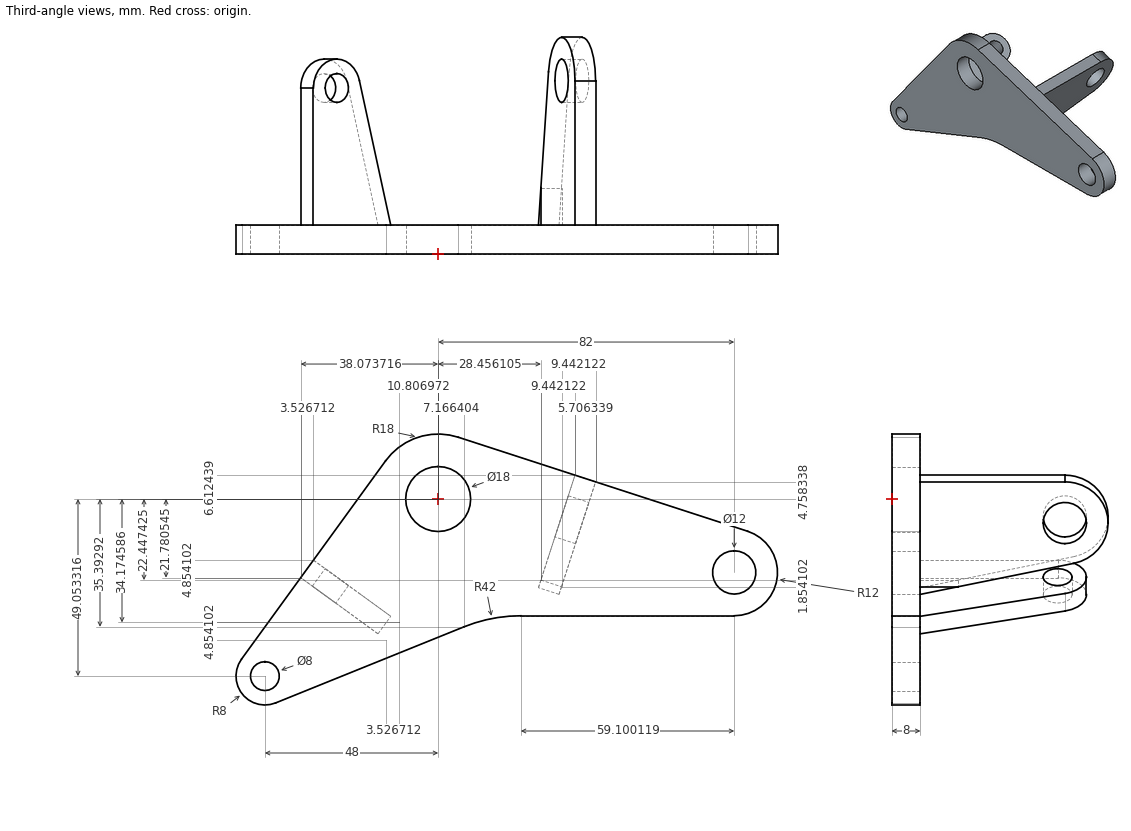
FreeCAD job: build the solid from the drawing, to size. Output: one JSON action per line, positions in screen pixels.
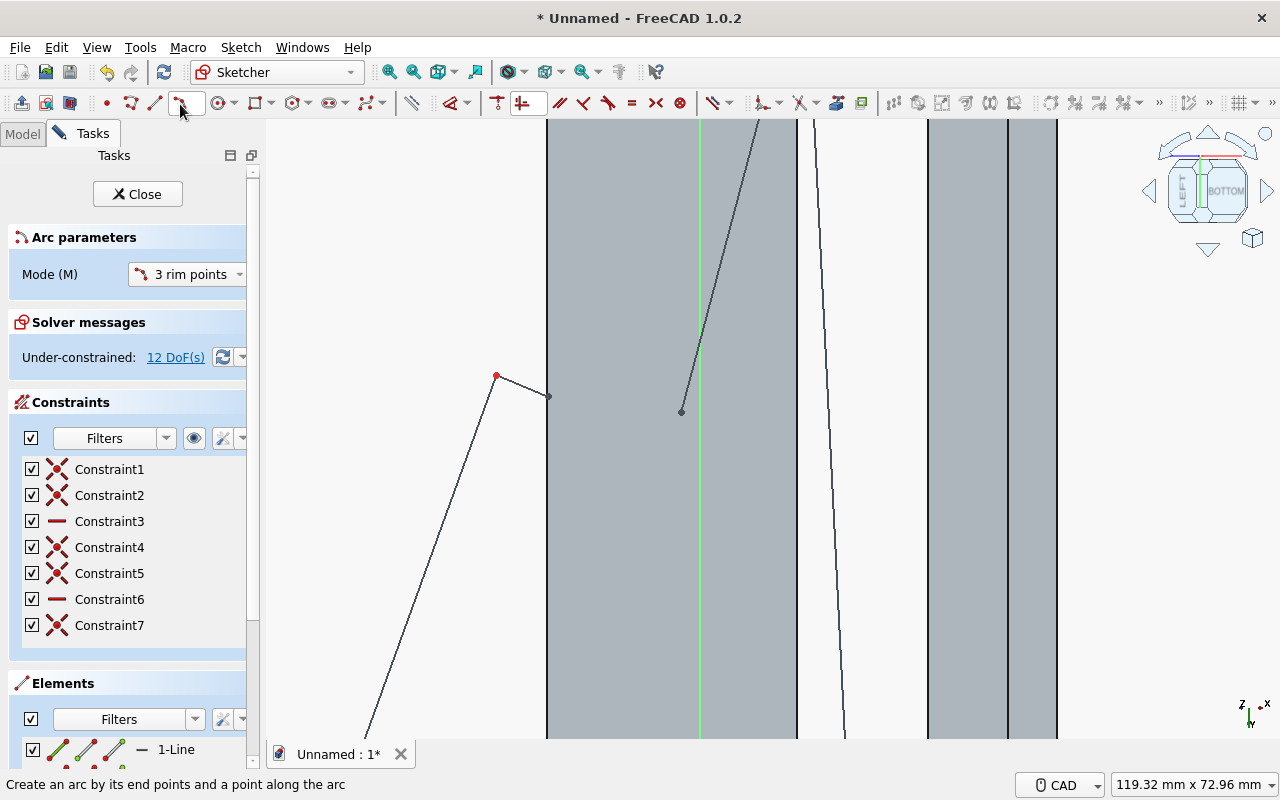
{"action": "left_click", "coordinate": [681, 413]}
{"action": "left_click", "coordinate": [548, 397]}
{"action": "left_click", "coordinate": [607, 462]}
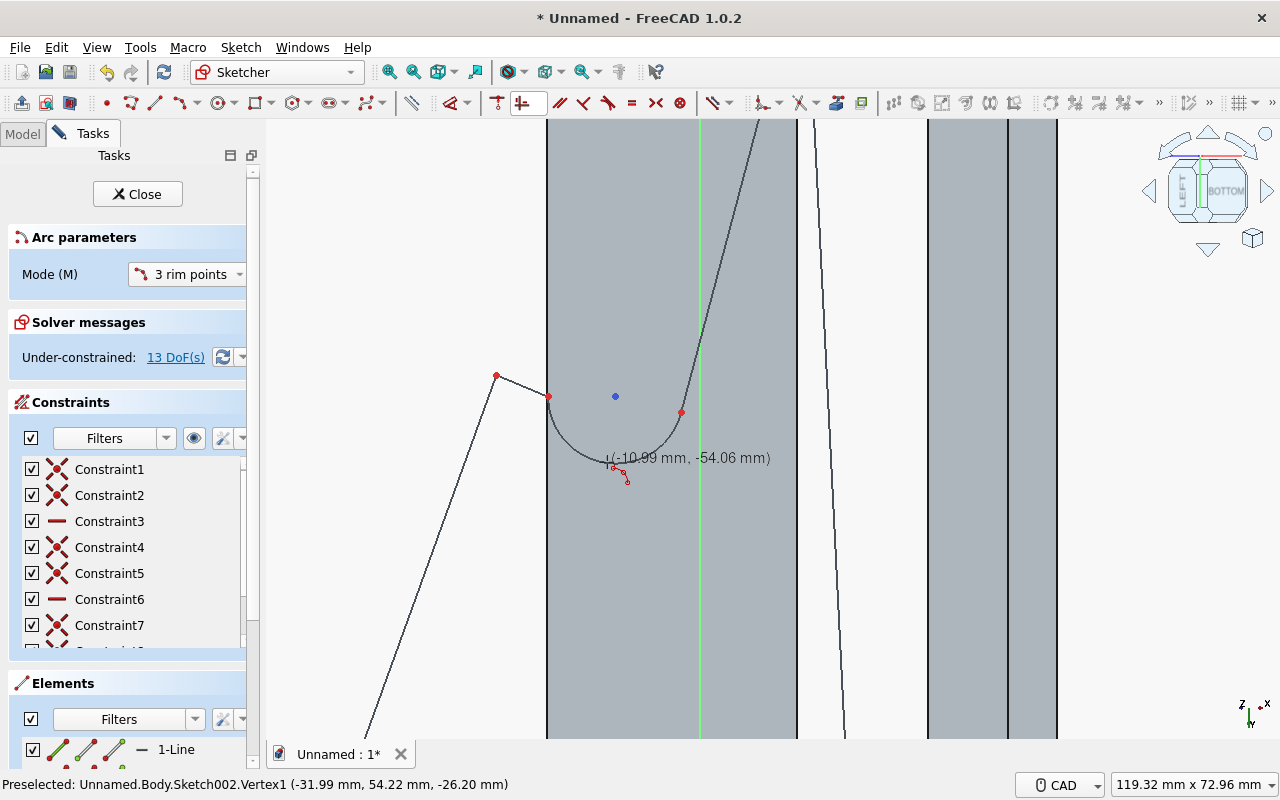
{"action": "left_click", "coordinate": [218, 104]}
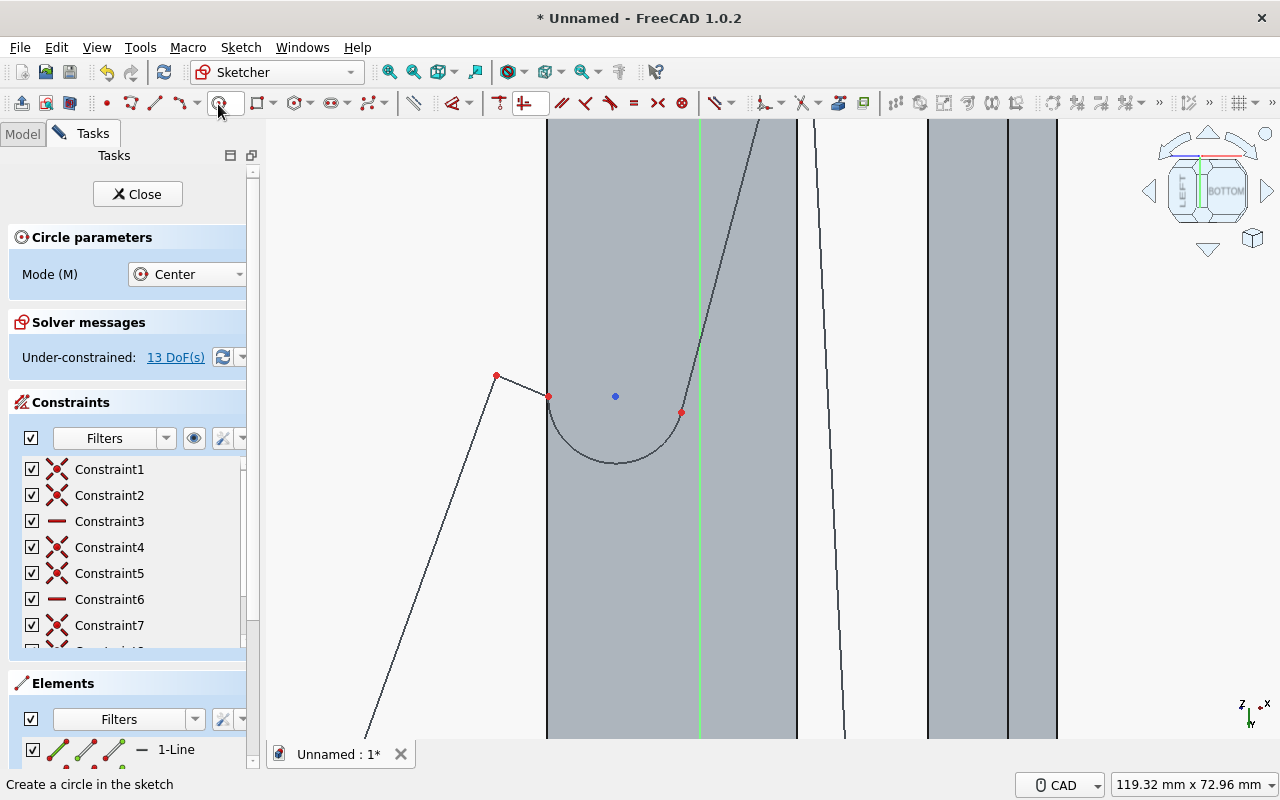
{"action": "left_click", "coordinate": [615, 394]}
{"action": "mouse_move", "coordinate": [639, 370]}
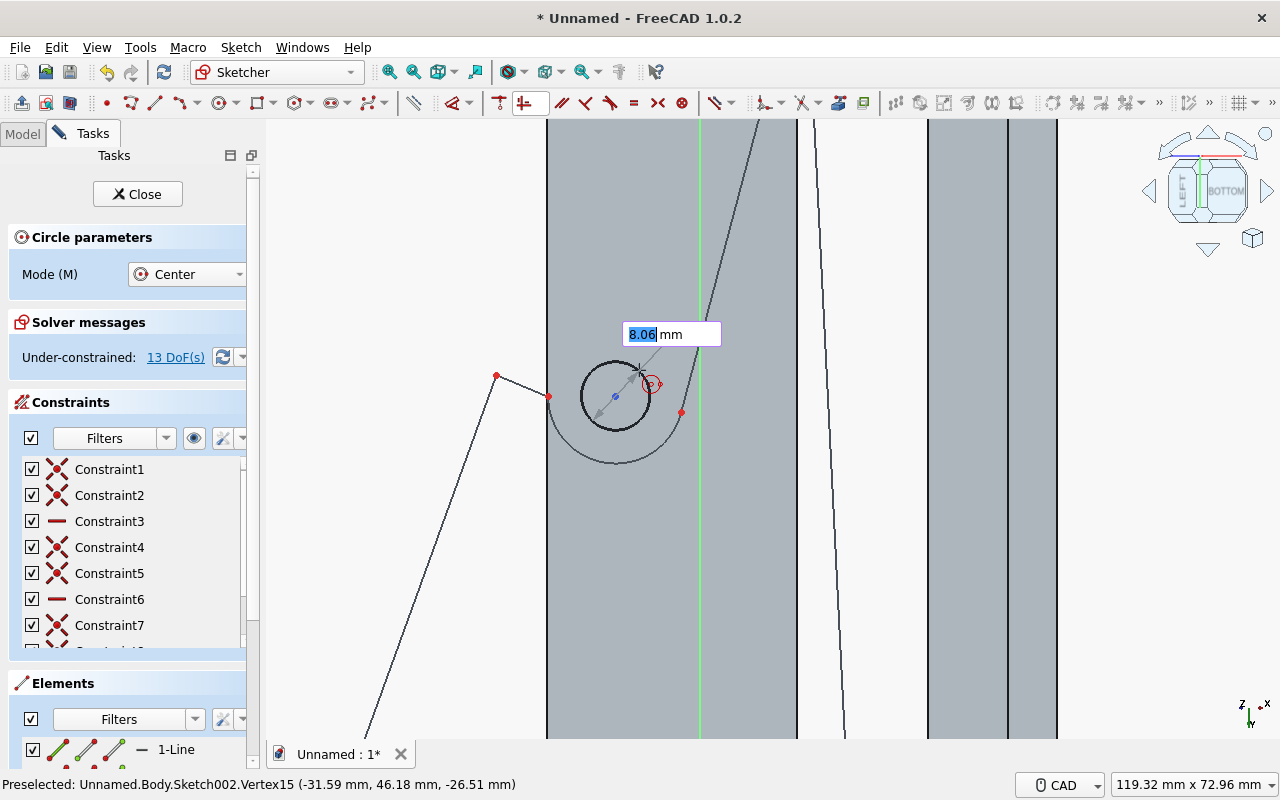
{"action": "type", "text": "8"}
{"action": "key", "text": "Return"}
{"action": "key", "text": "Escape"}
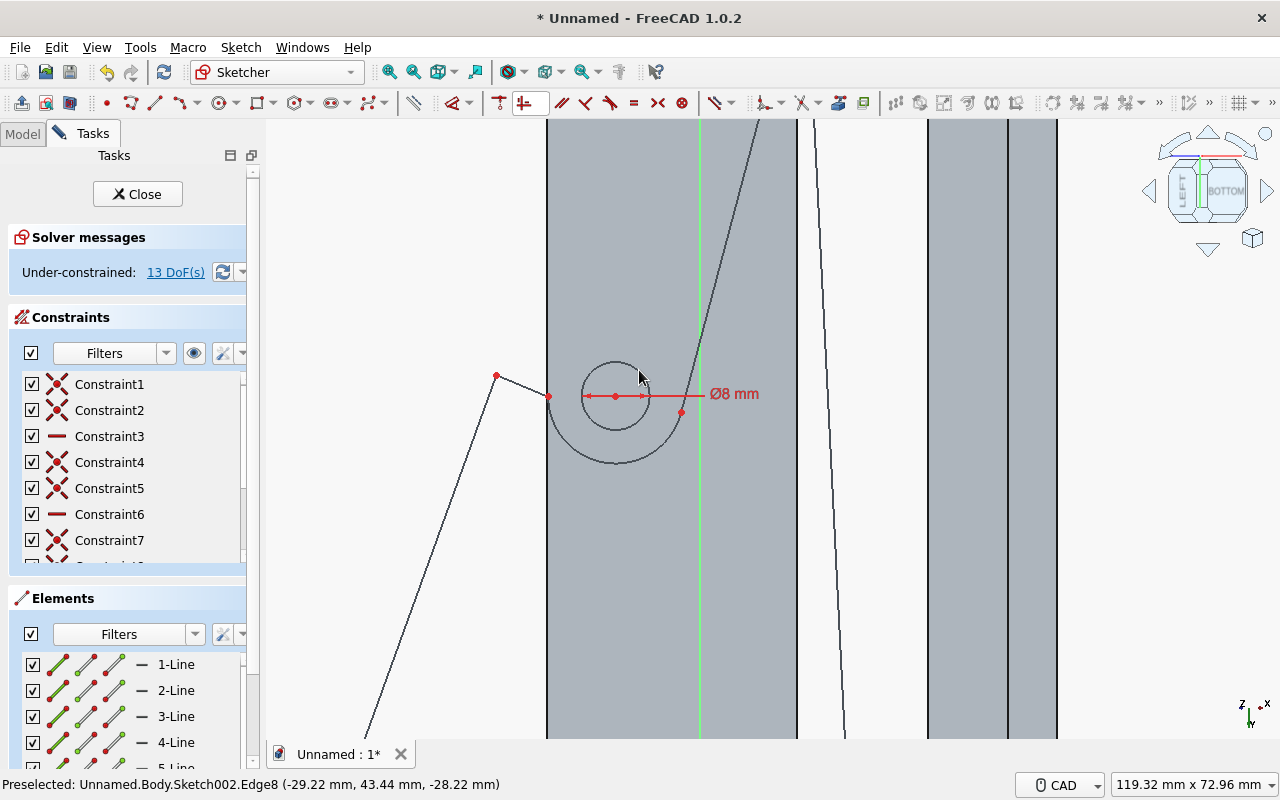
{"action": "left_click", "coordinate": [744, 175]}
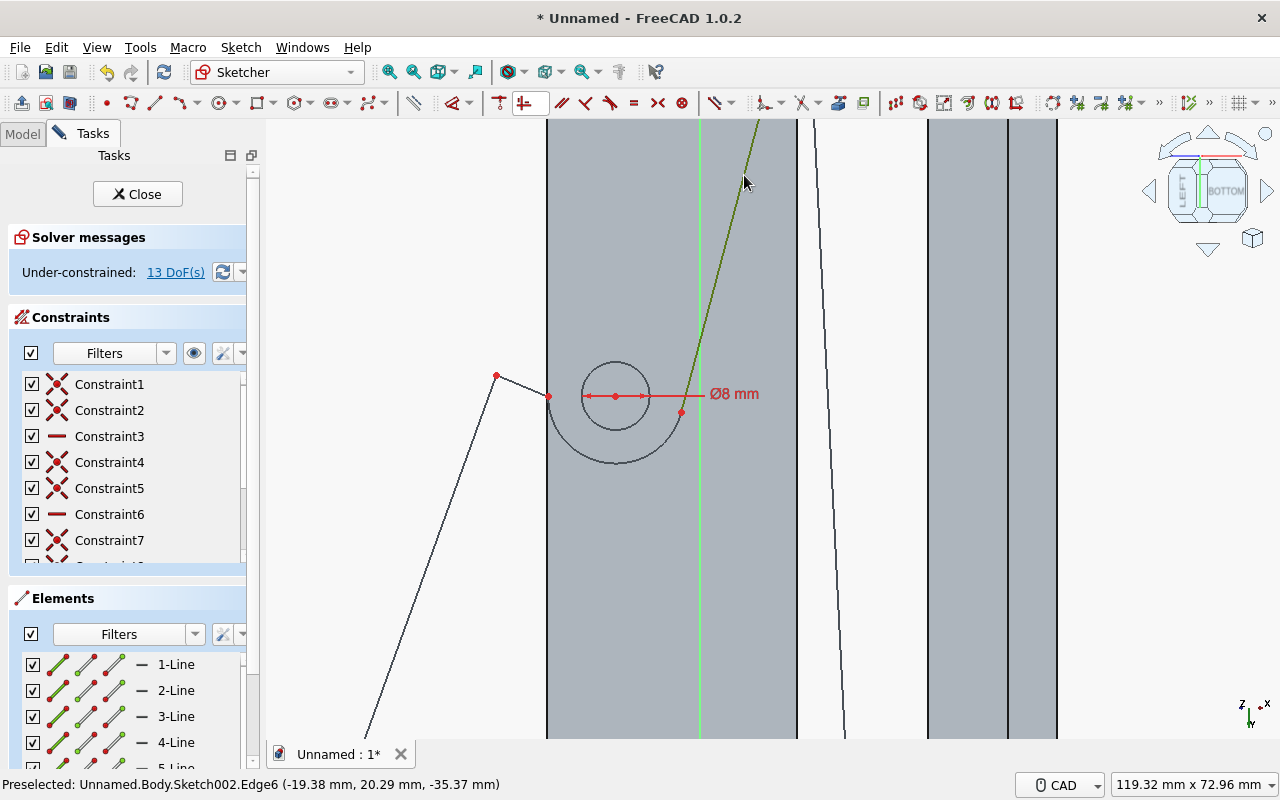
{"action": "left_click", "coordinate": [572, 448]}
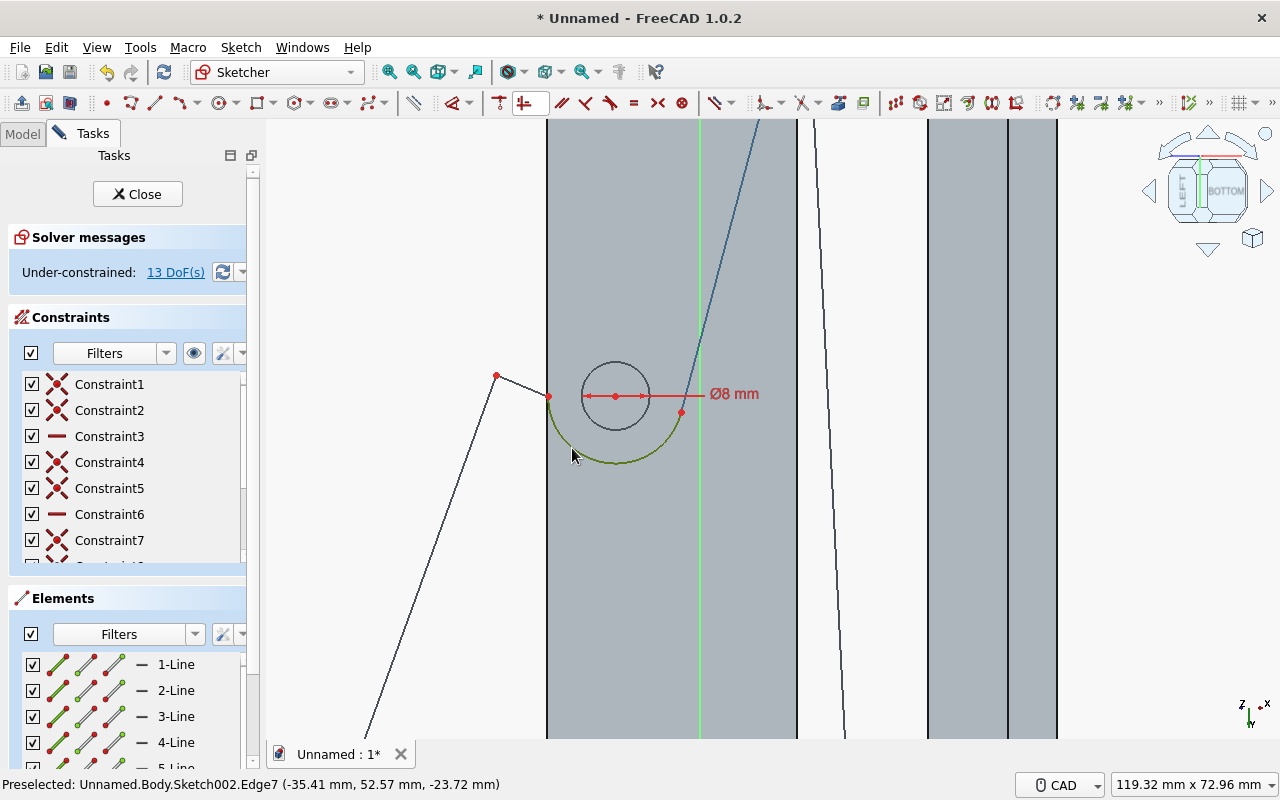
{"action": "left_click", "coordinate": [610, 104]}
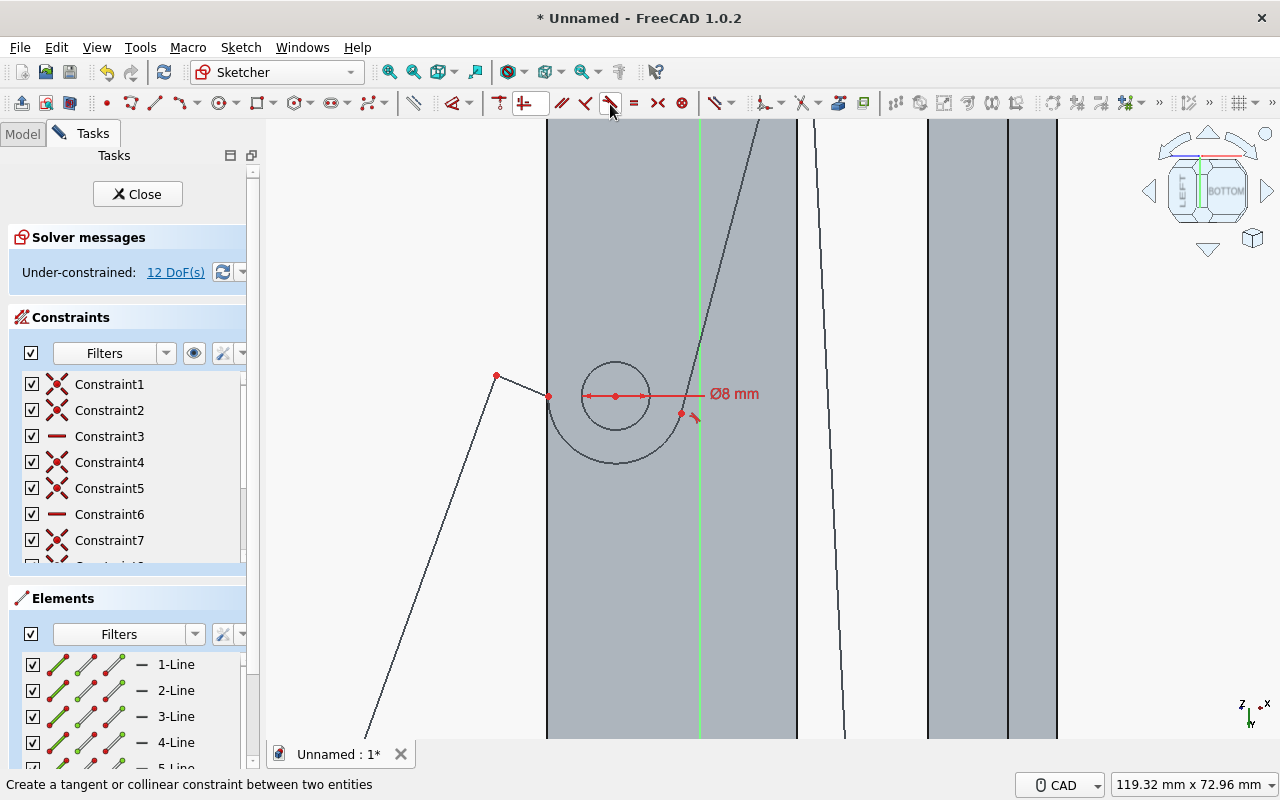
{"action": "left_click", "coordinate": [452, 104]}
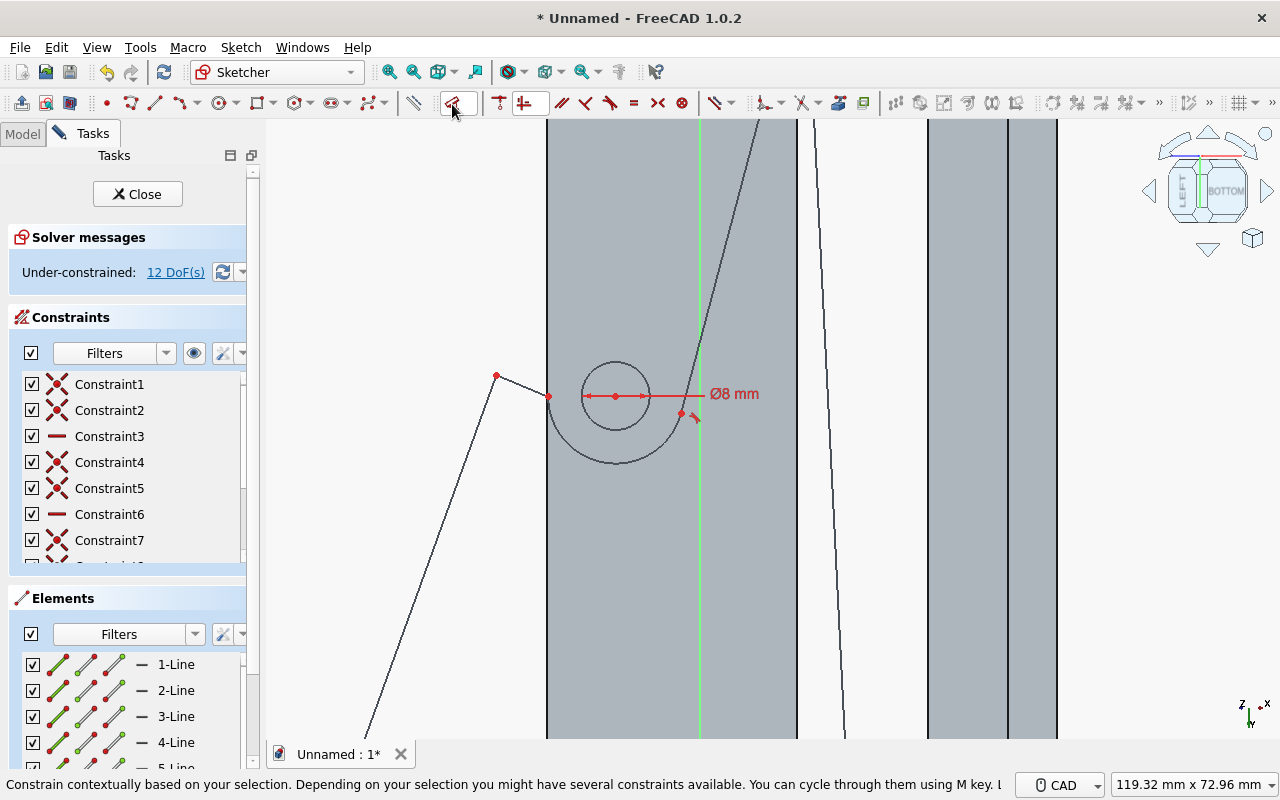
{"action": "left_click", "coordinate": [572, 448]}
{"action": "left_click", "coordinate": [551, 473]}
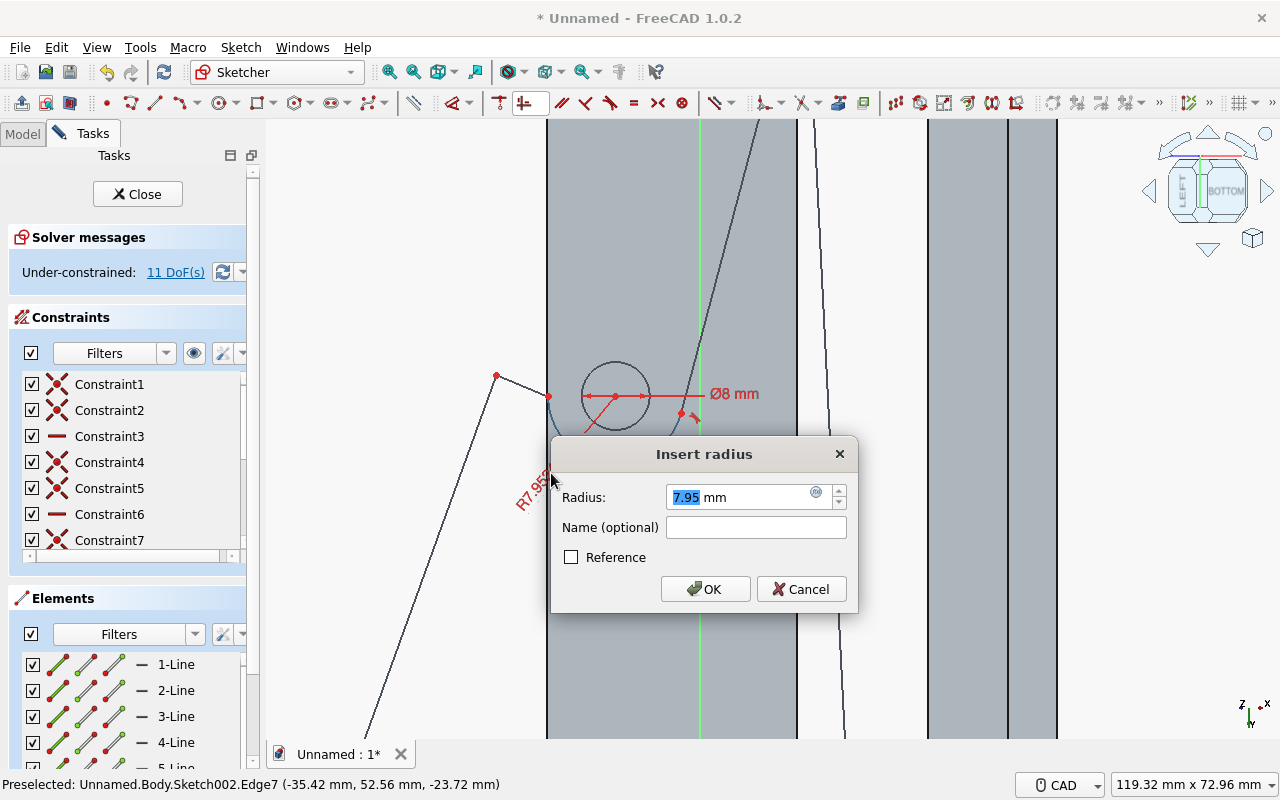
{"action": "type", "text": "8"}
{"action": "key", "text": "Return"}